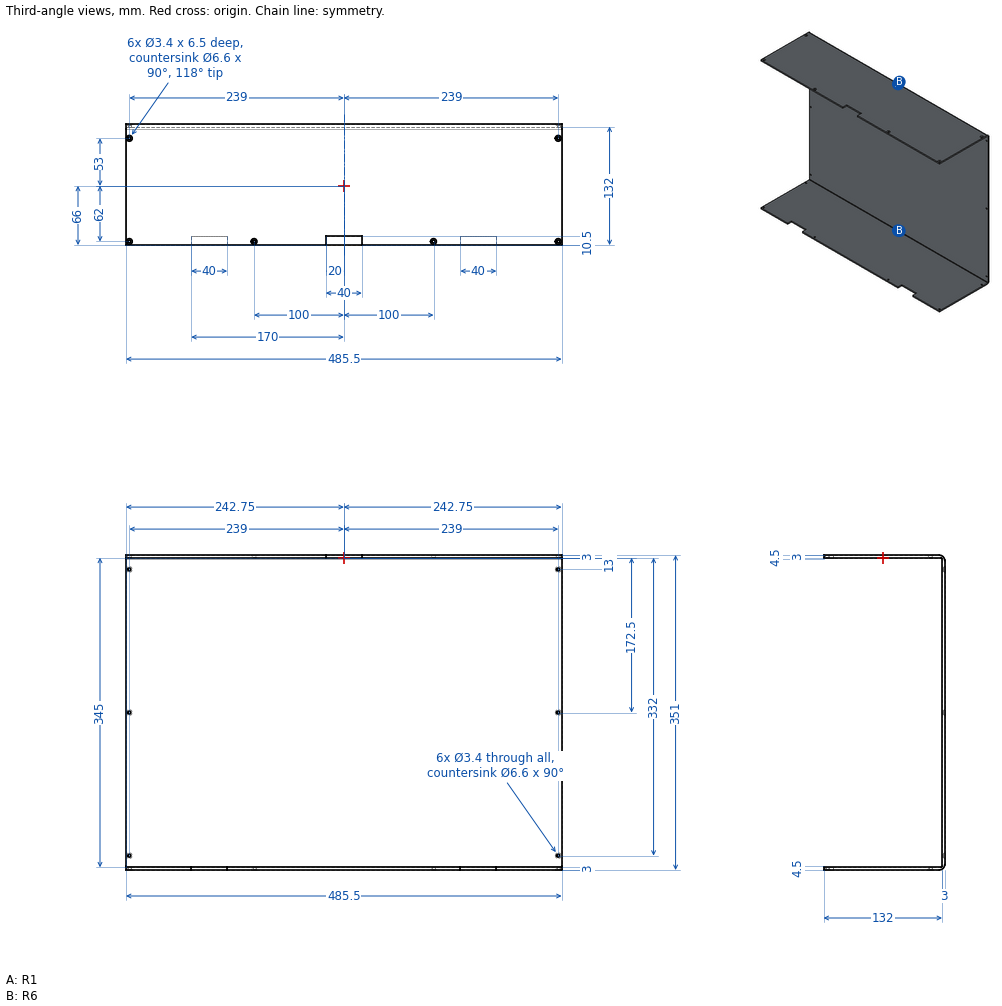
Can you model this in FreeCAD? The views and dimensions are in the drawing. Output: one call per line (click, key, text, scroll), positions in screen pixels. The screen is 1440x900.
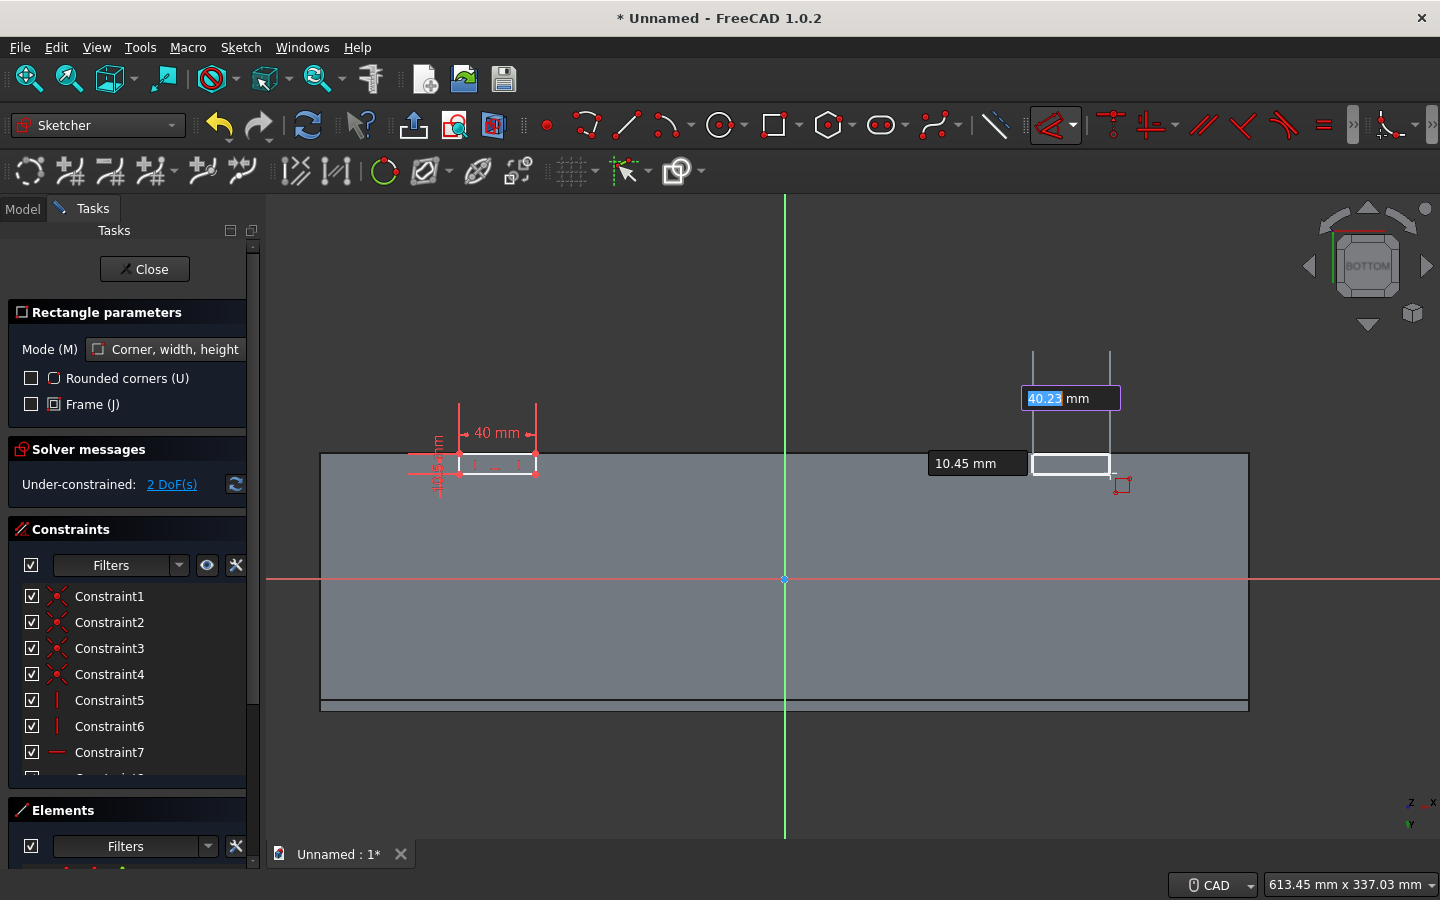
text(40)
key(Tab)
text(10.5)
key(Return)
key(Escape)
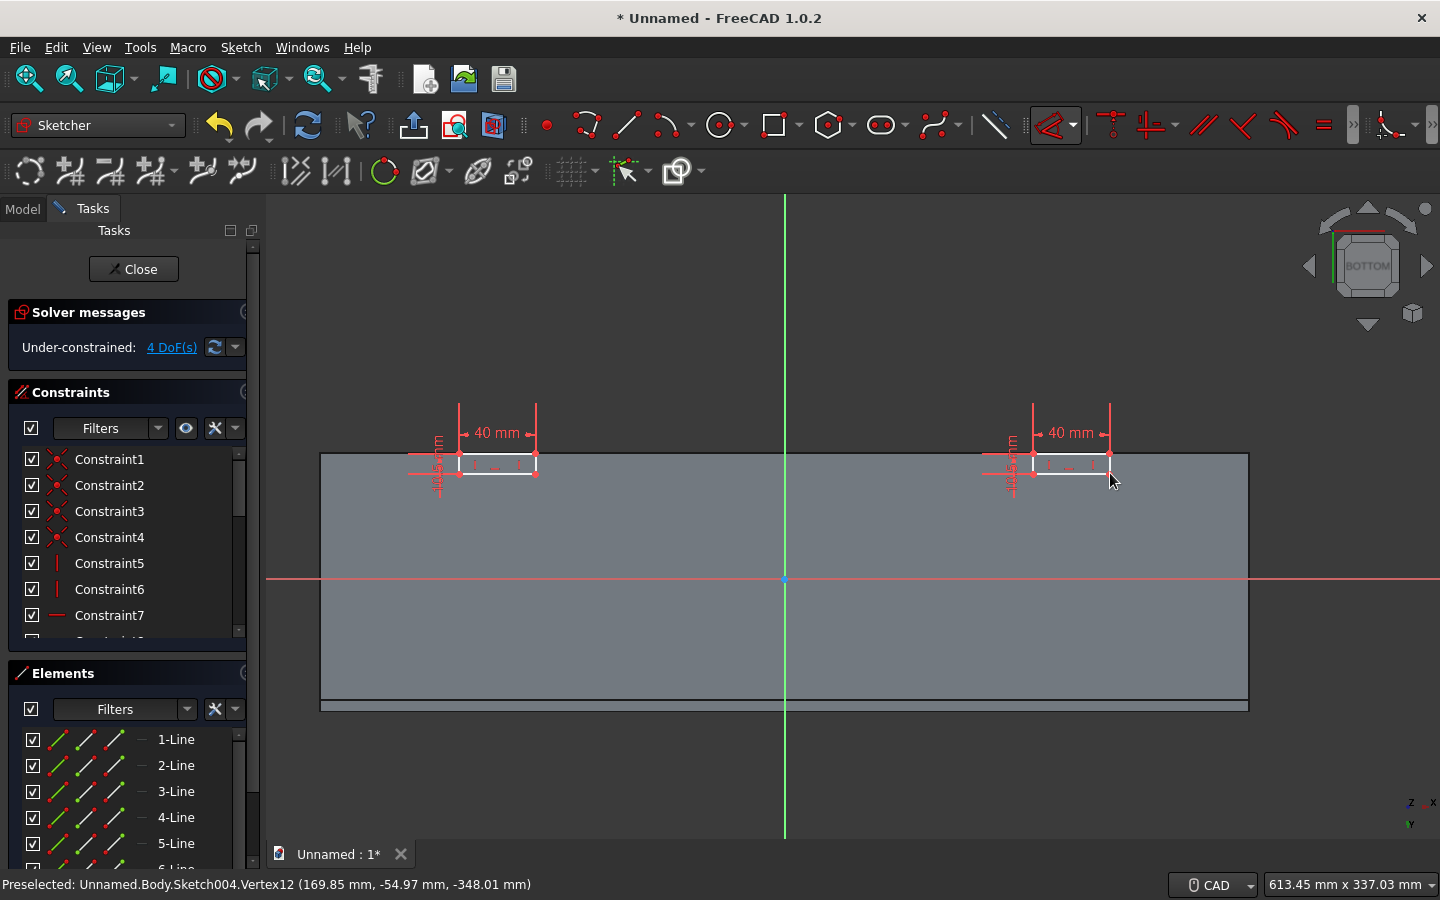
click(536, 454)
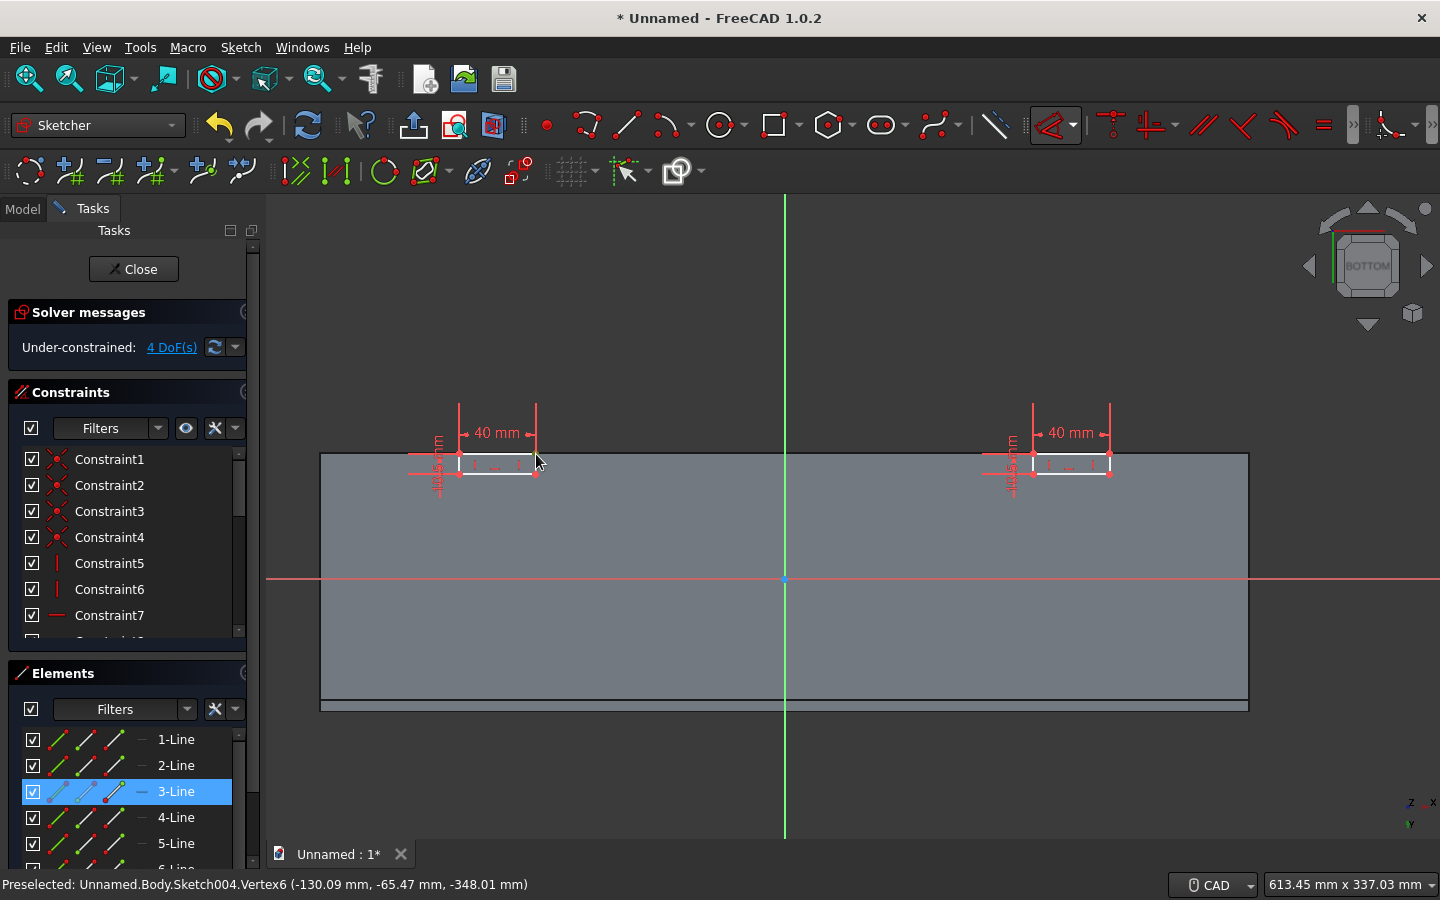
click(1033, 454)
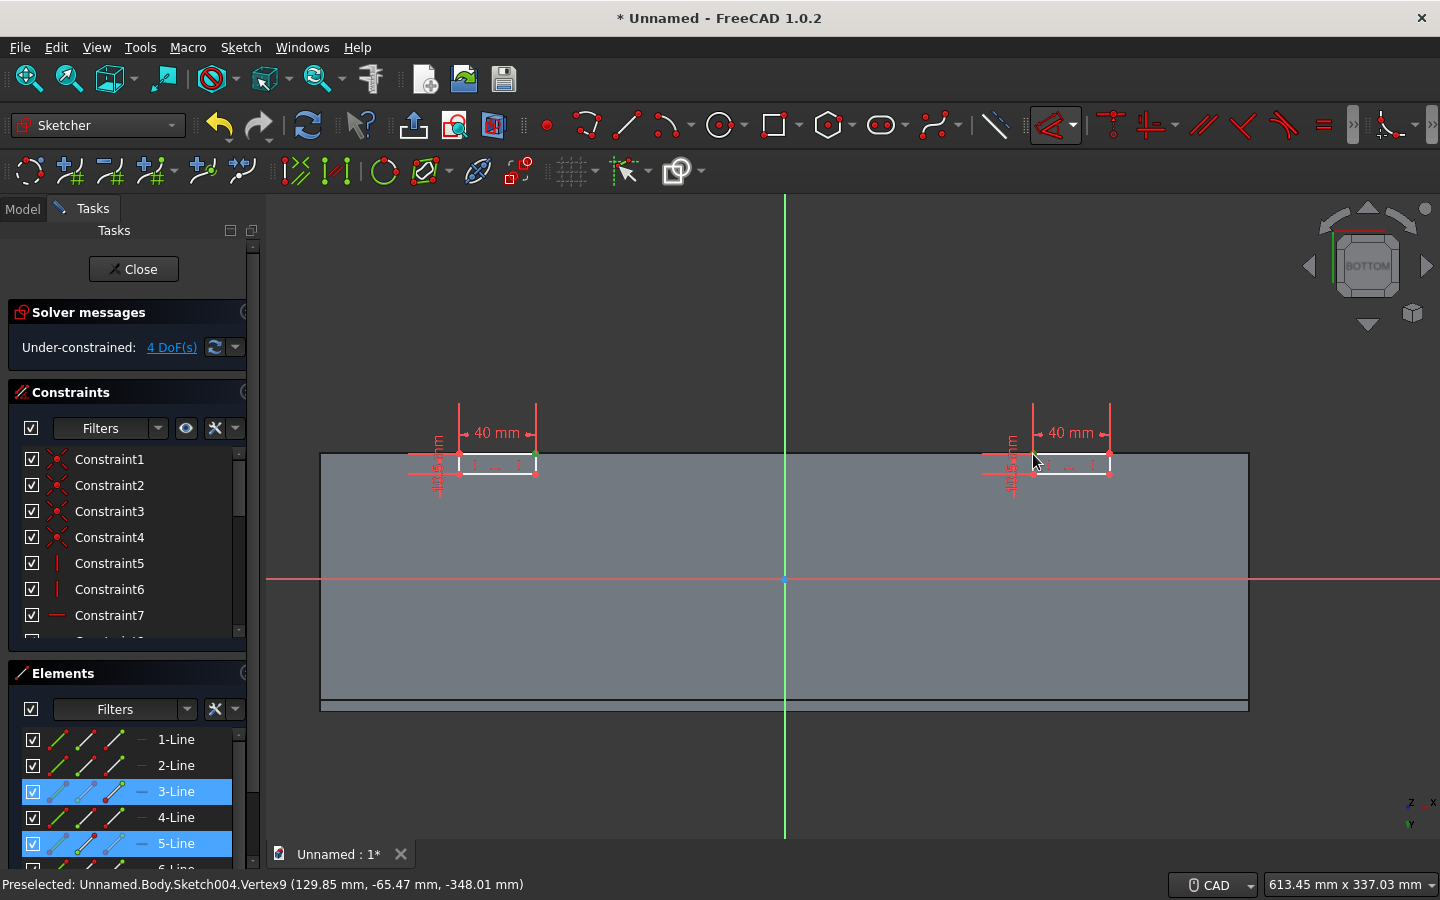
click(785, 769)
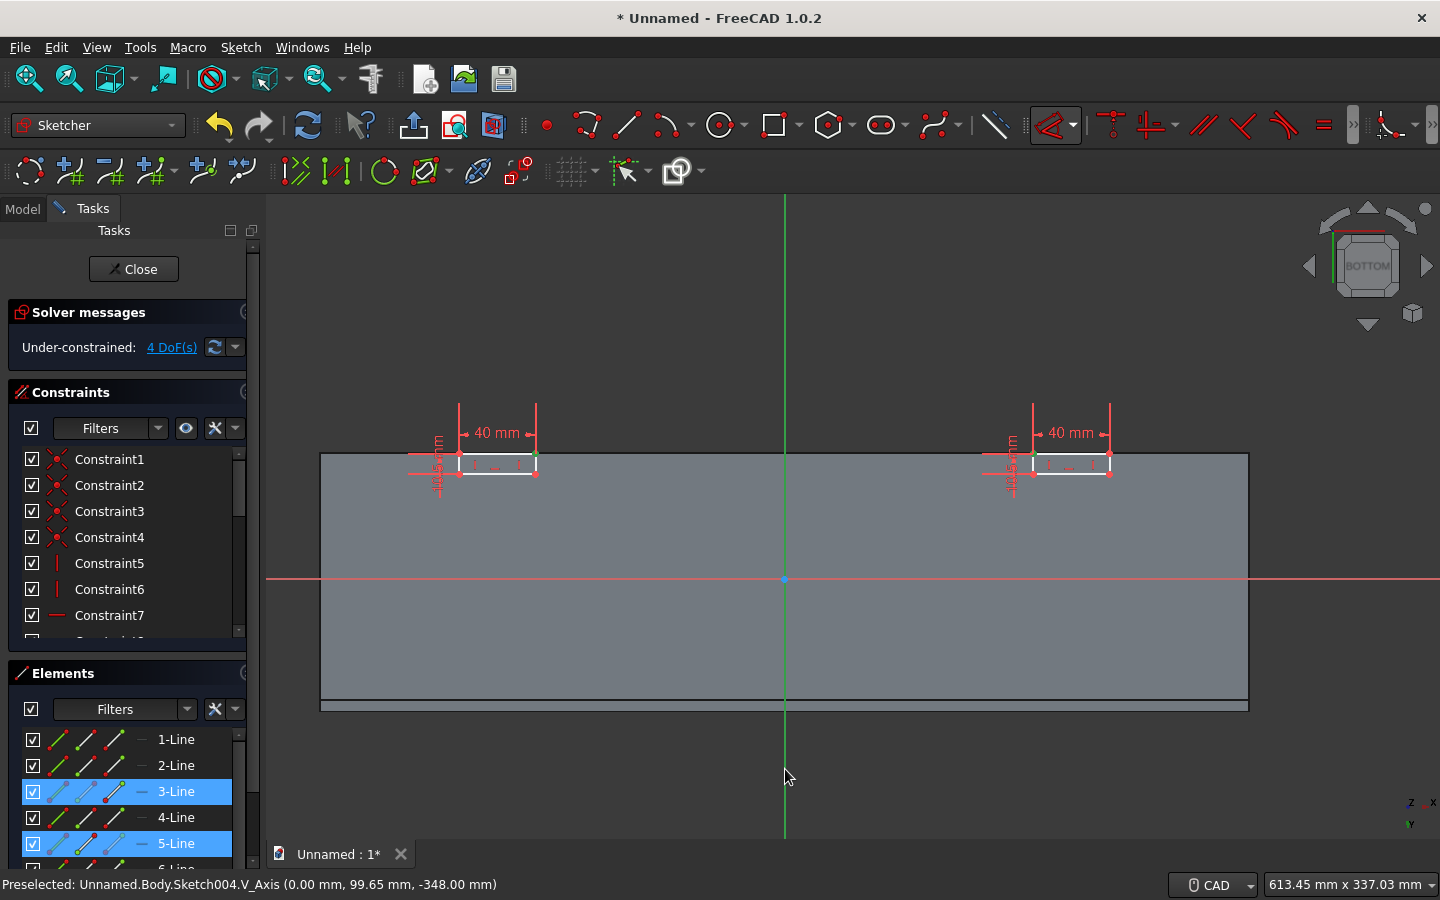
key(s)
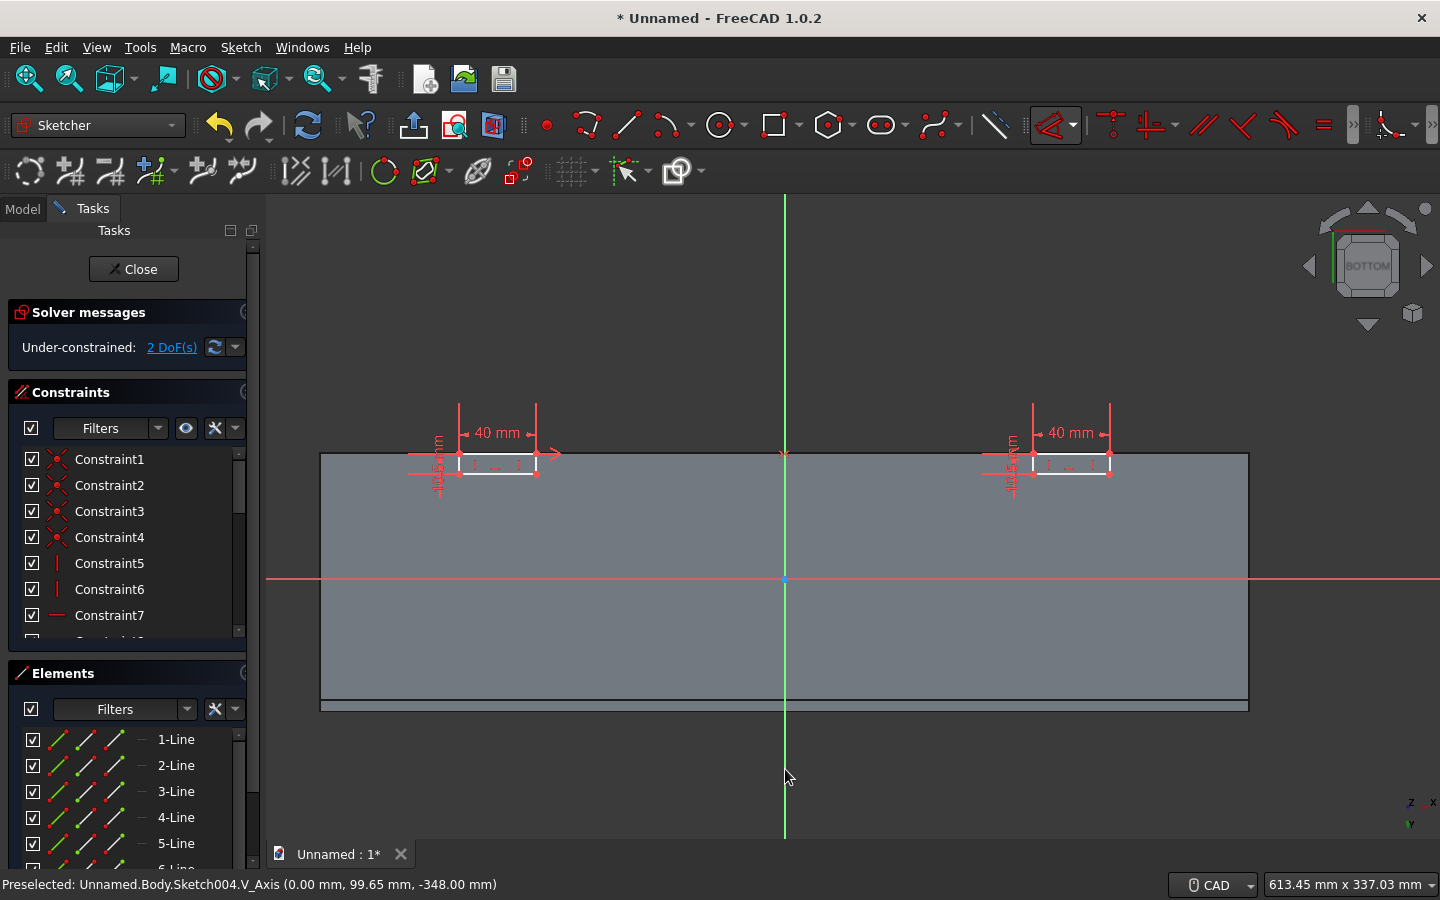
click(459, 454)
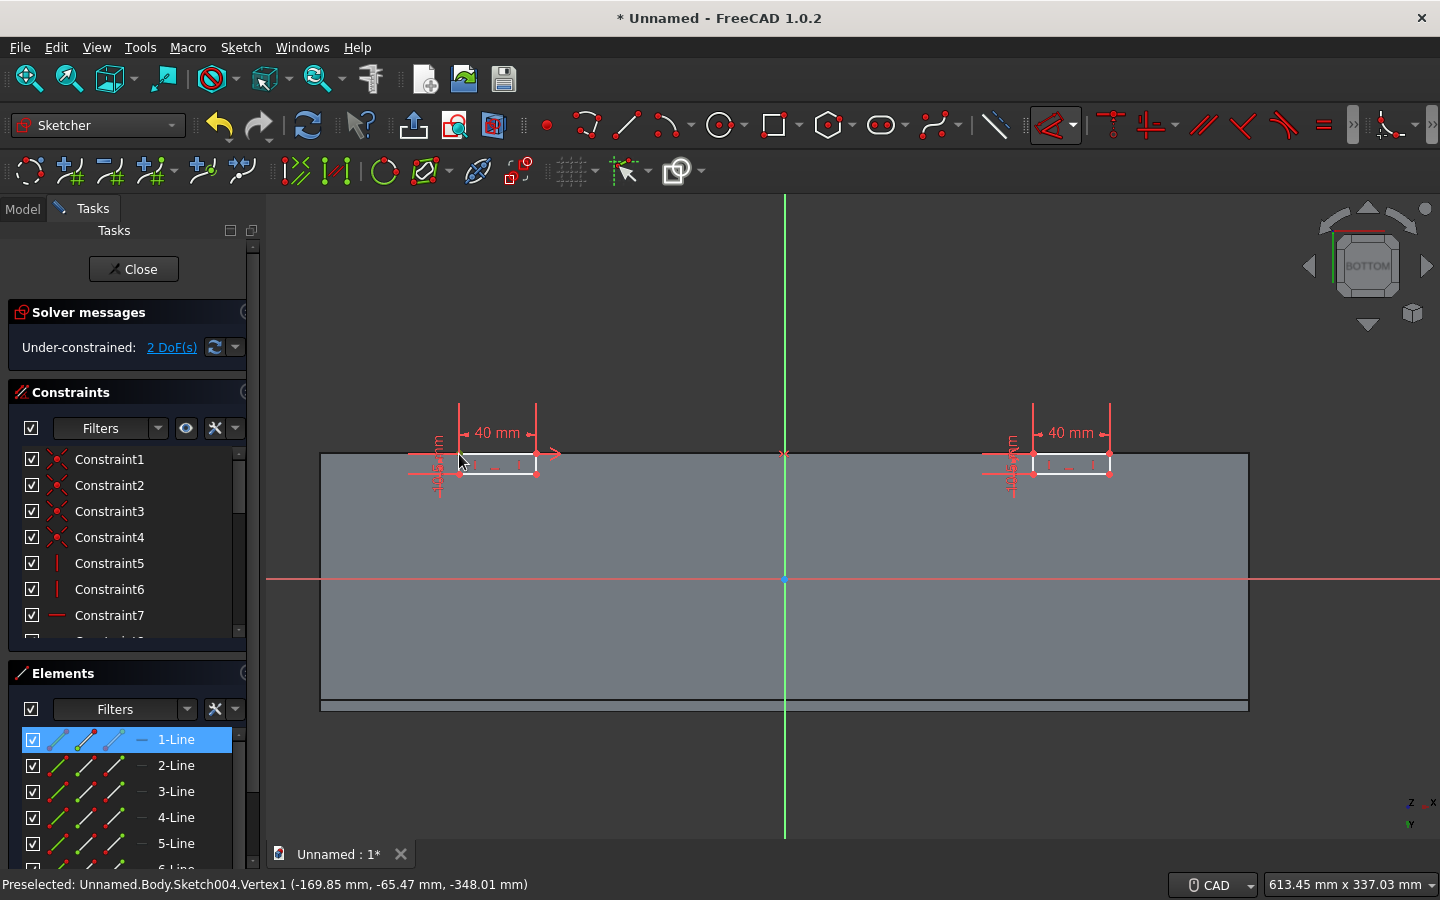
click(1076, 126)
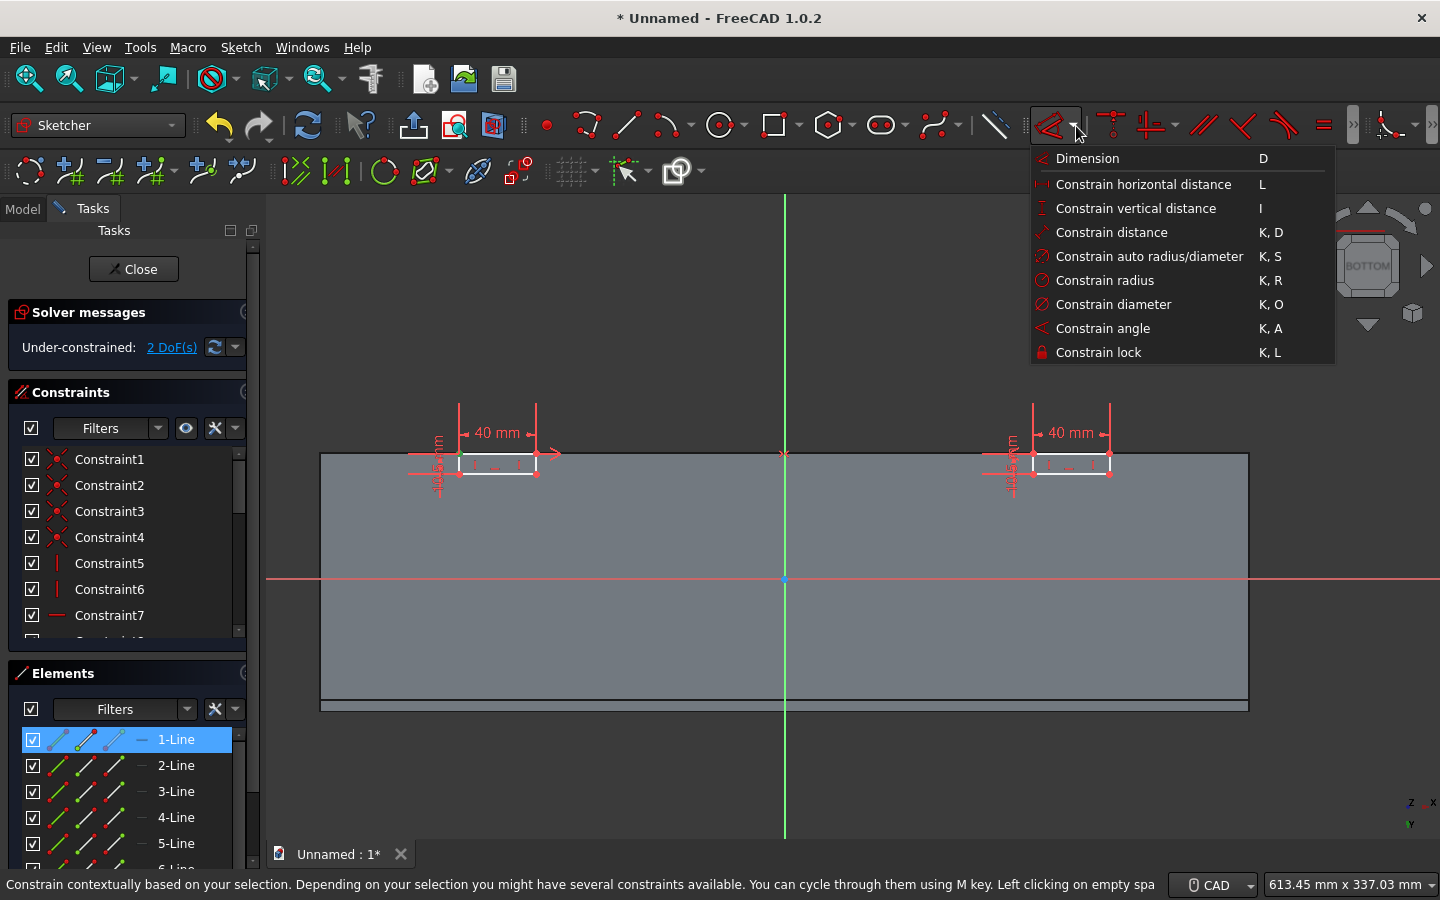
click(1183, 208)